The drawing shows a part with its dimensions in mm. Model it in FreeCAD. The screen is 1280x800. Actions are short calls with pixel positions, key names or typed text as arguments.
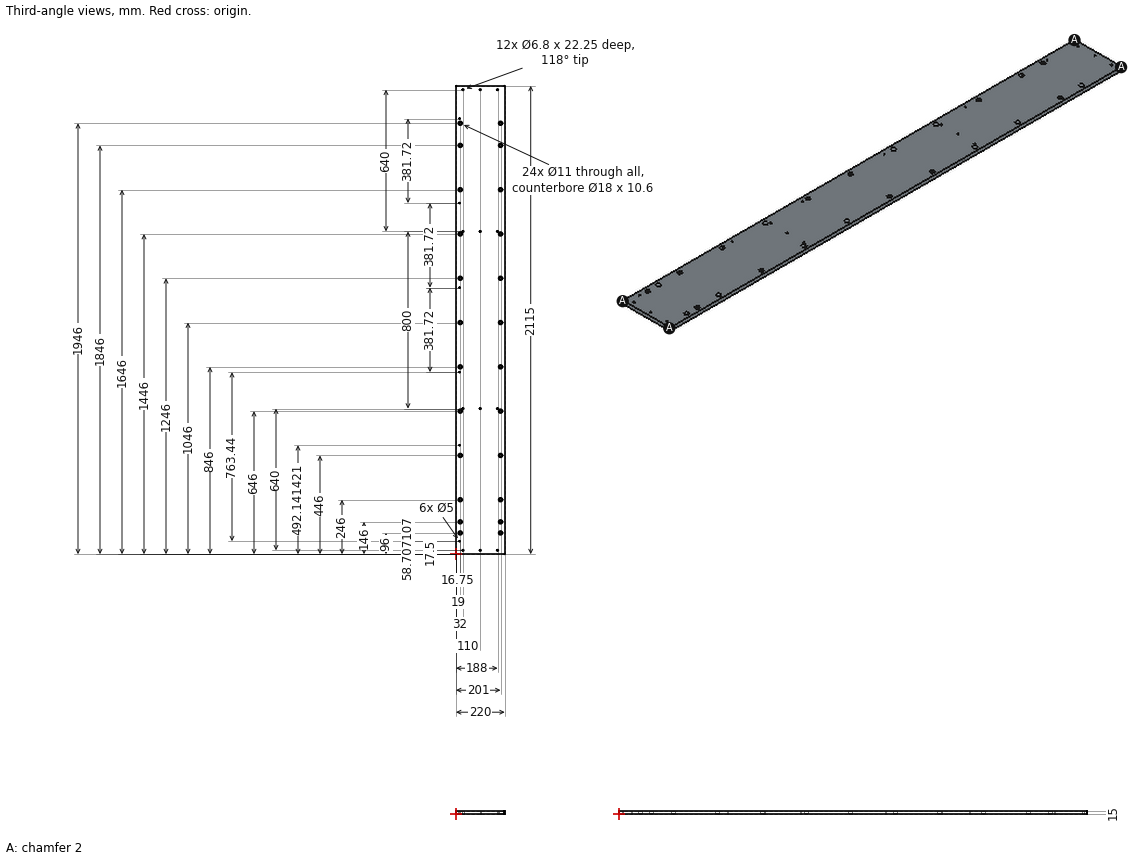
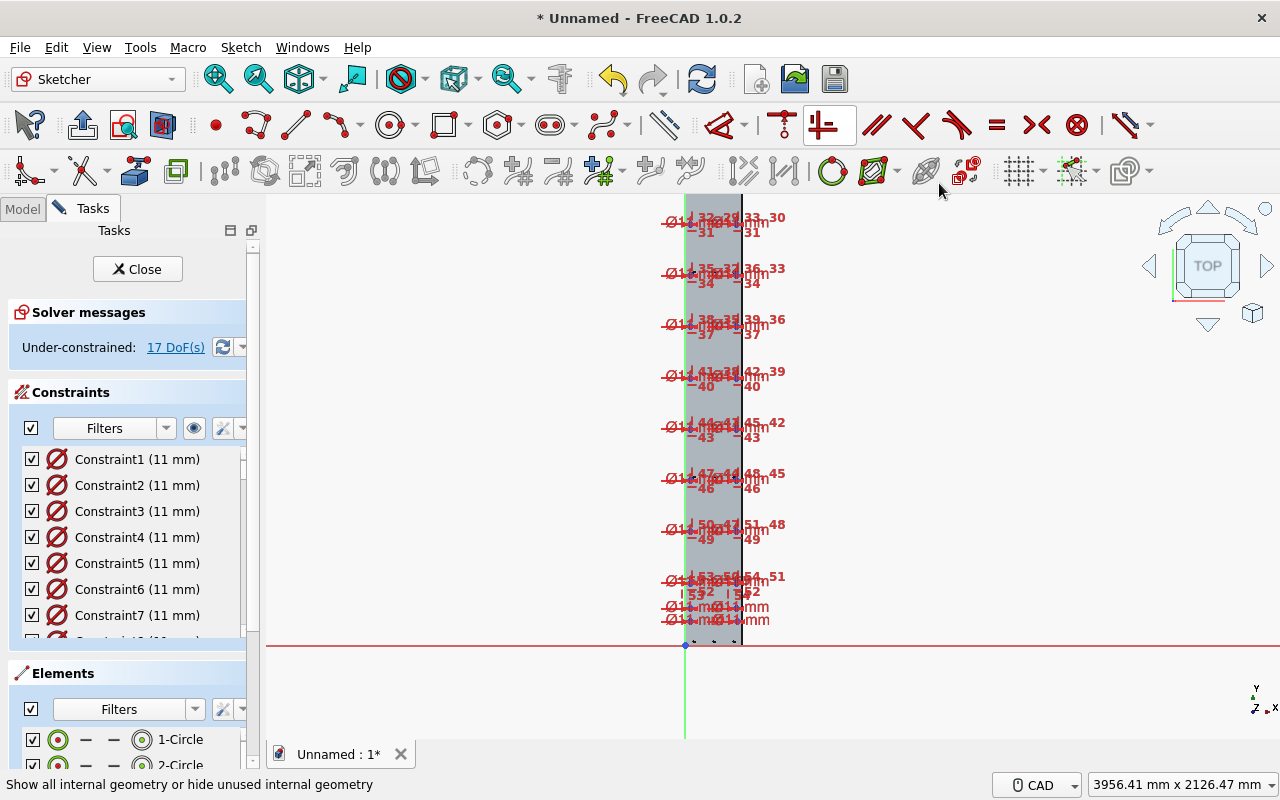
click(690, 609)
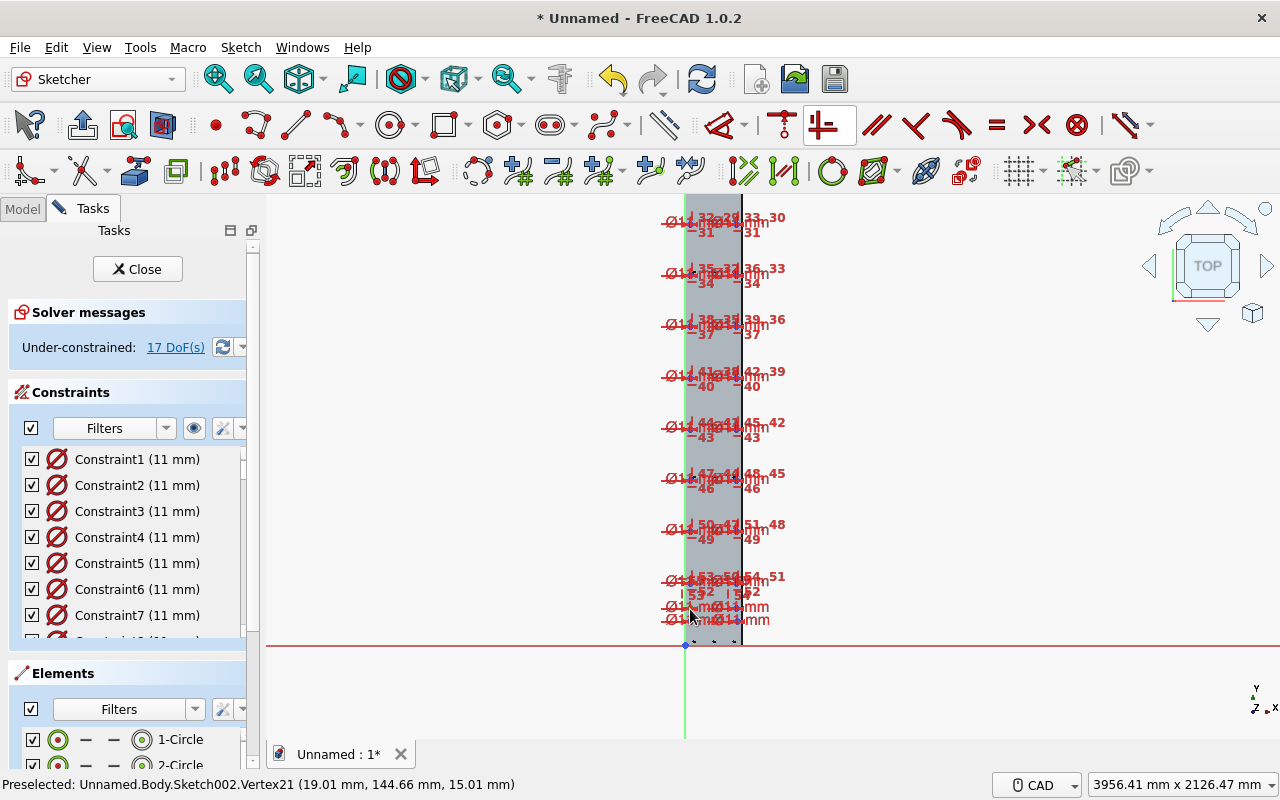
click(690, 622)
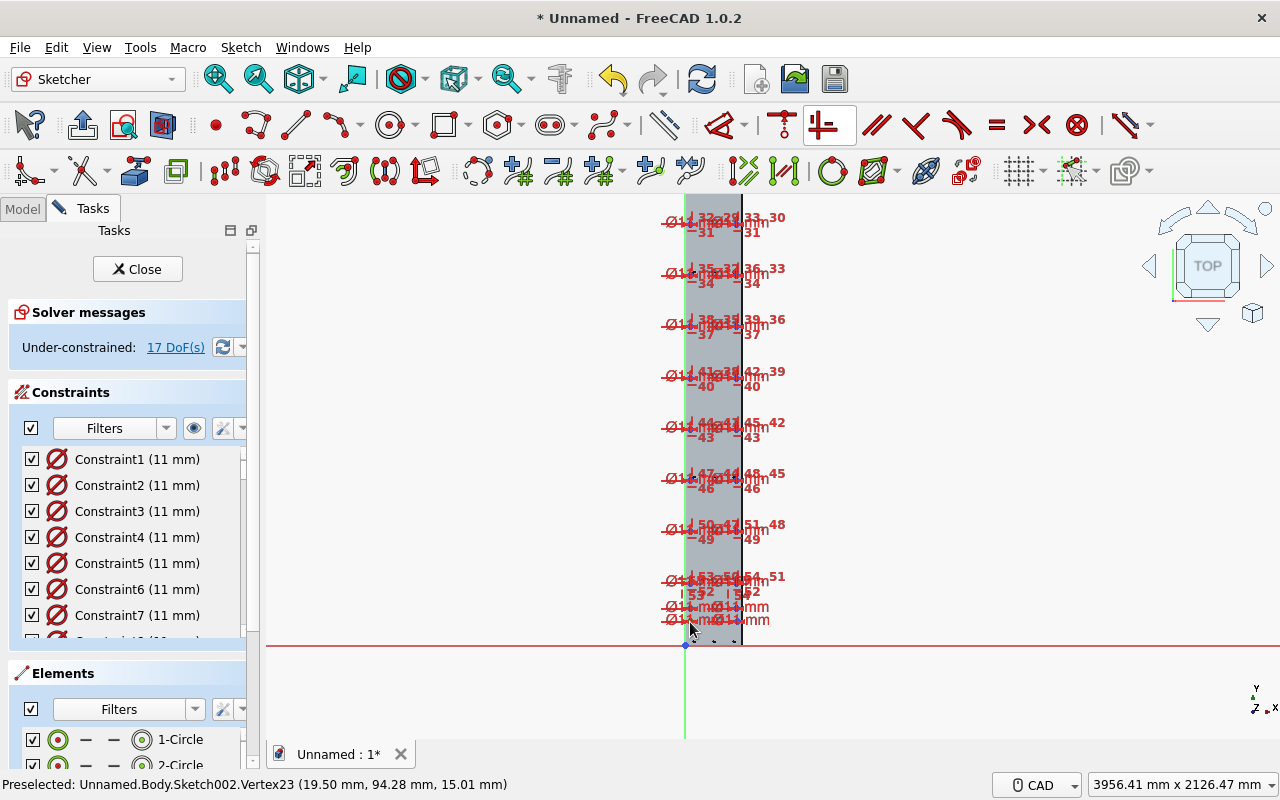
key(v)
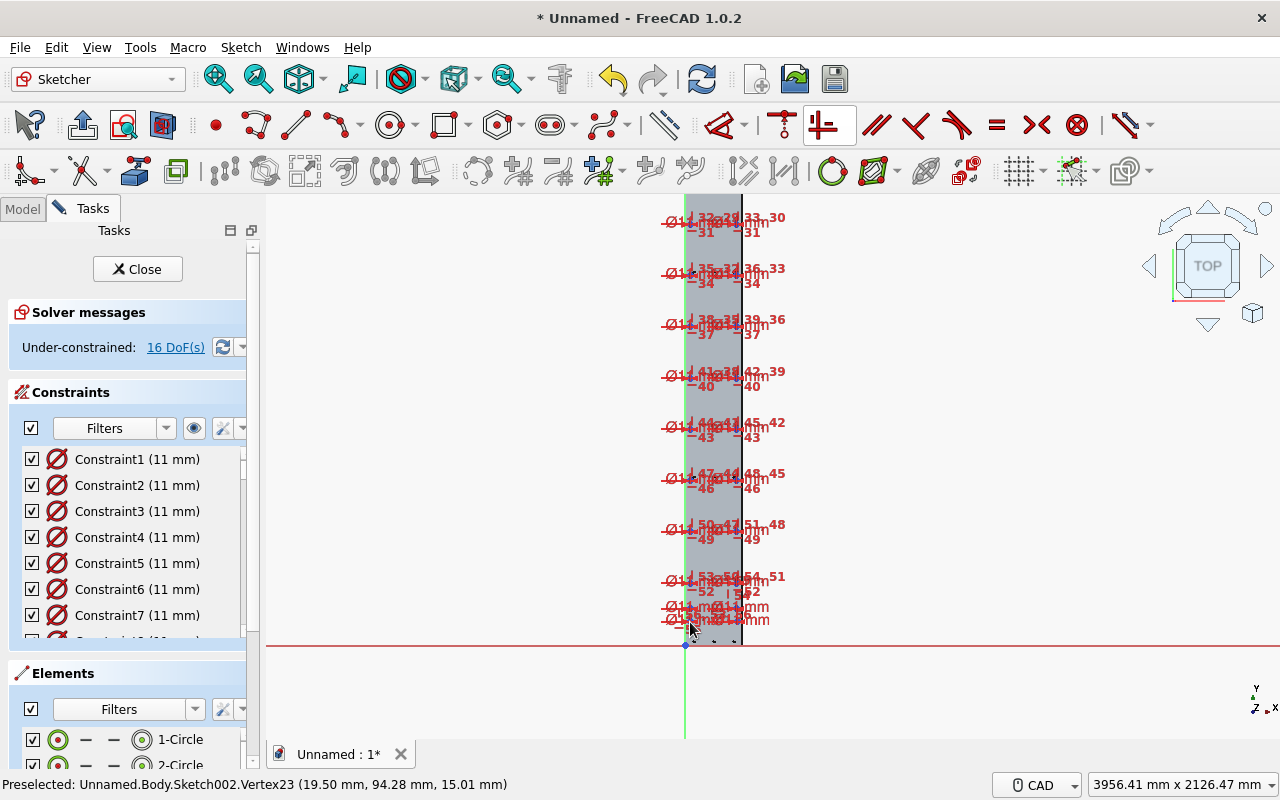
scroll(736, 609, up, 4)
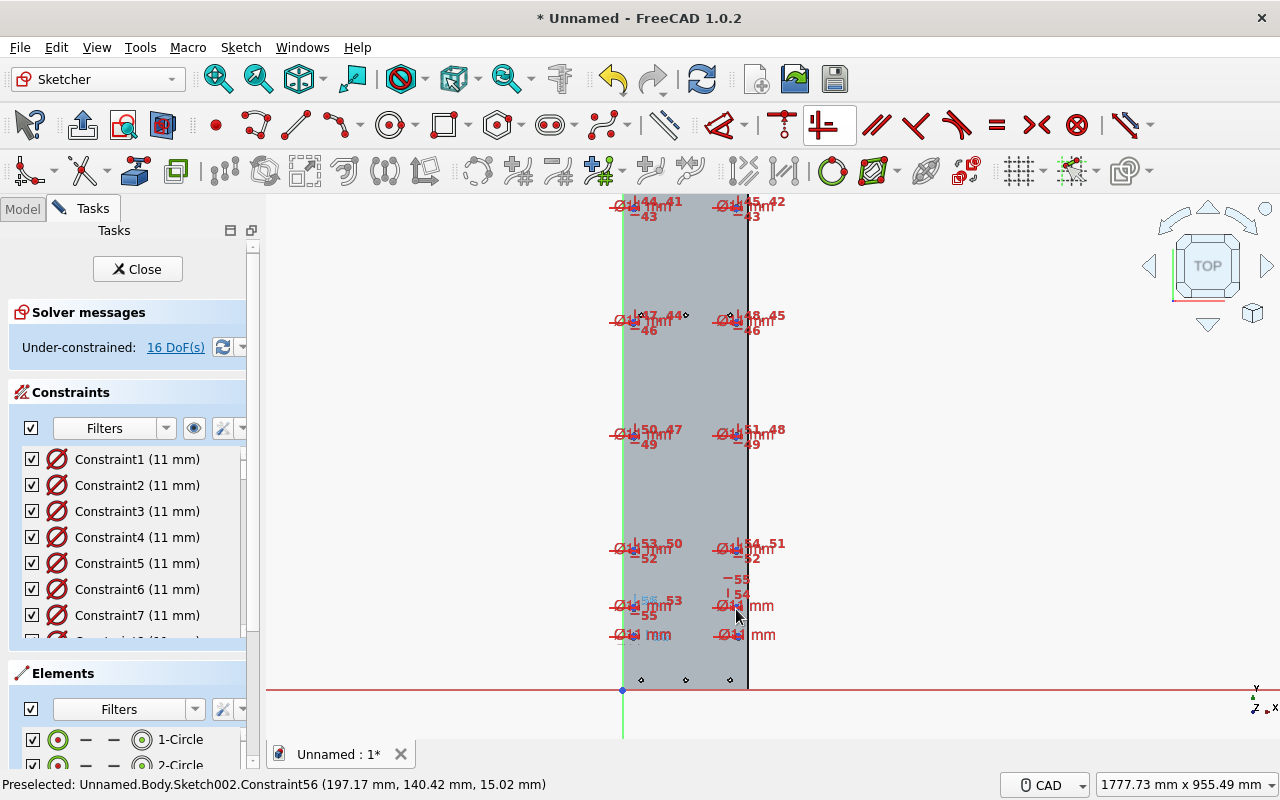
click(737, 608)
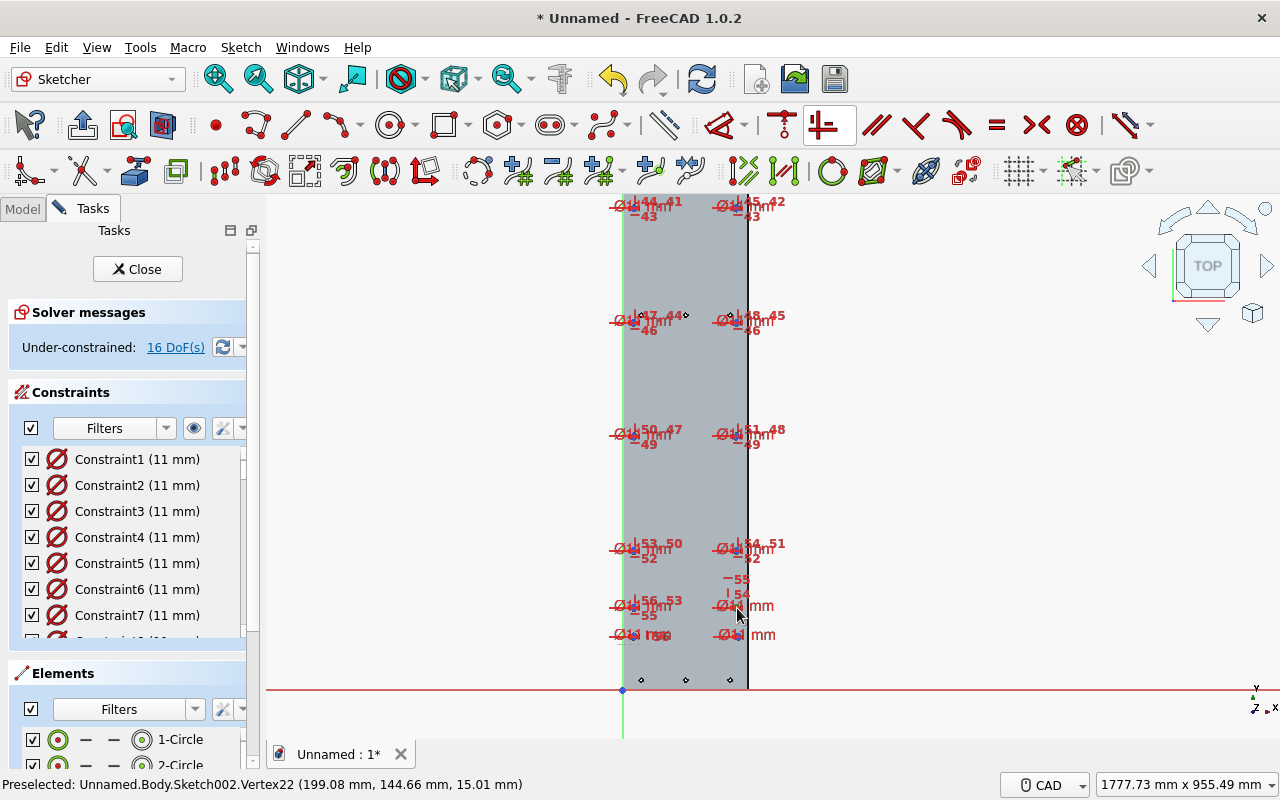
click(738, 637)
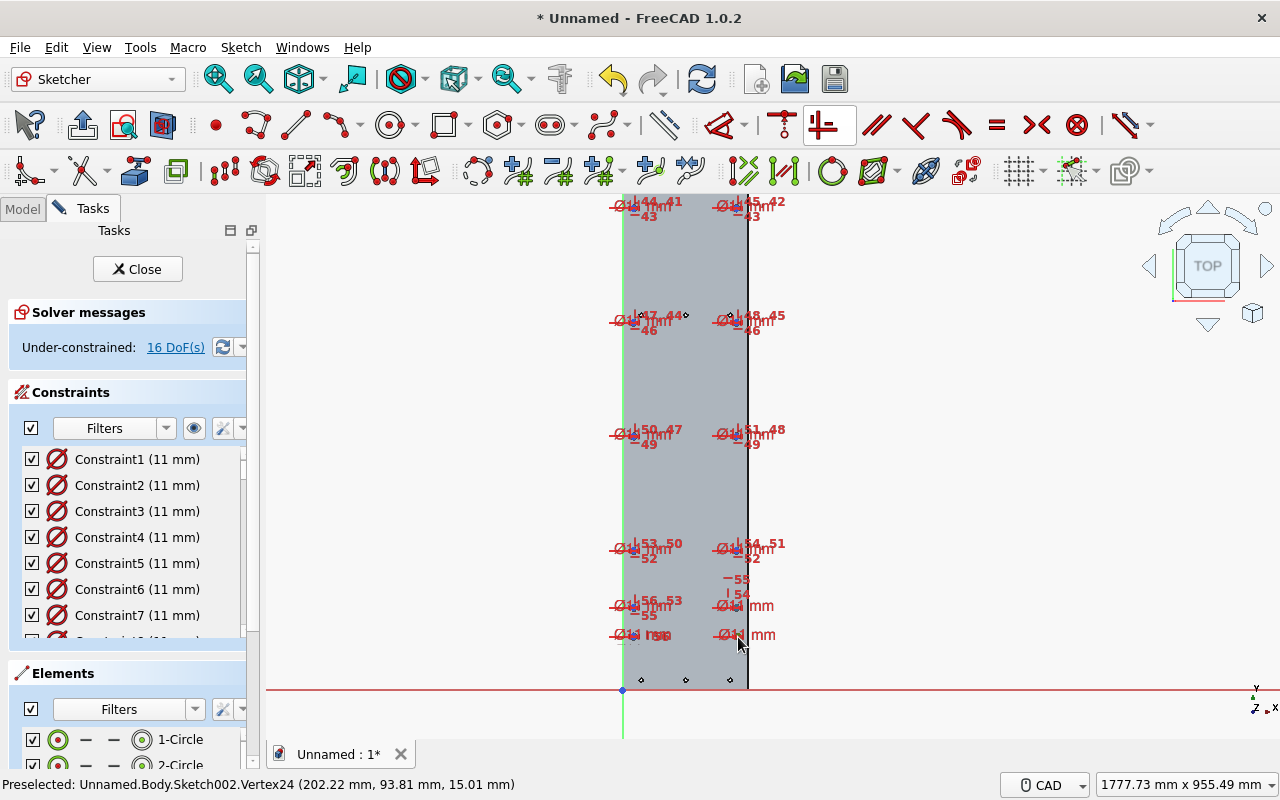
key(v)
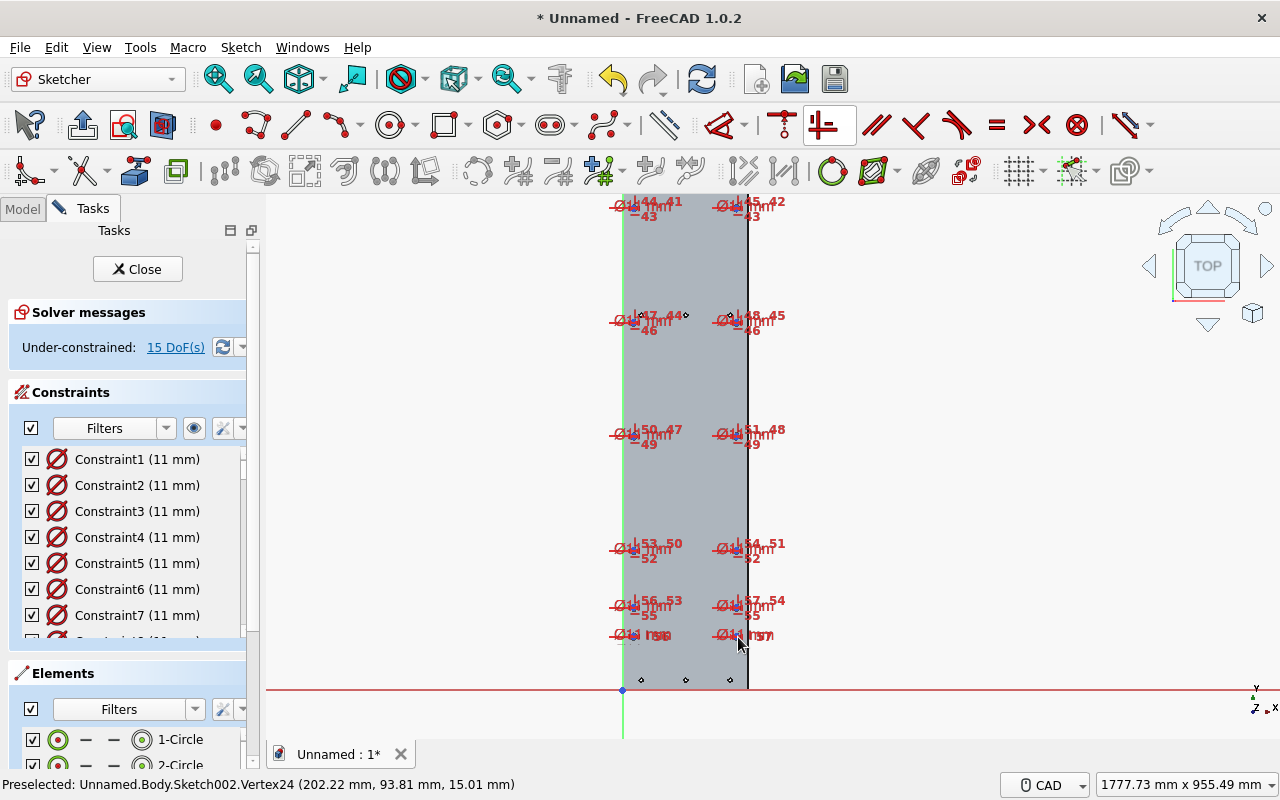
click(634, 637)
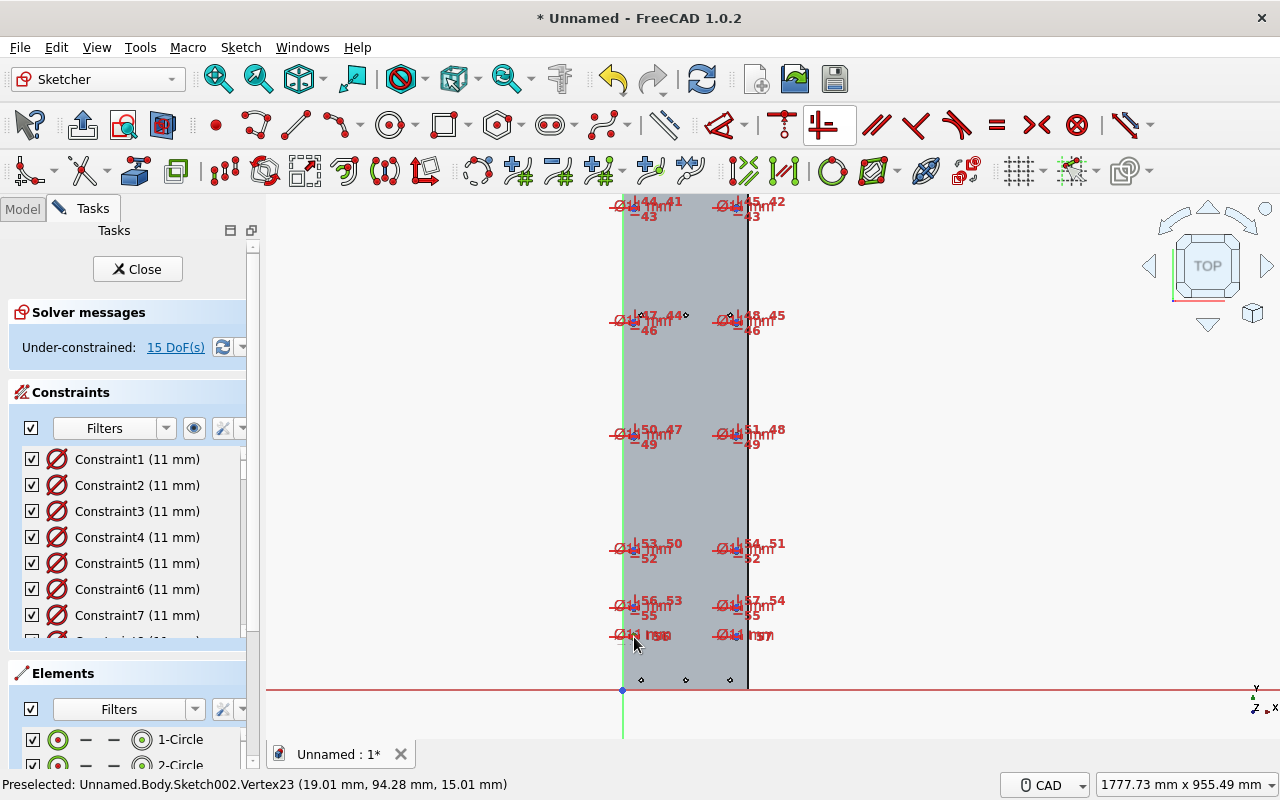
click(737, 637)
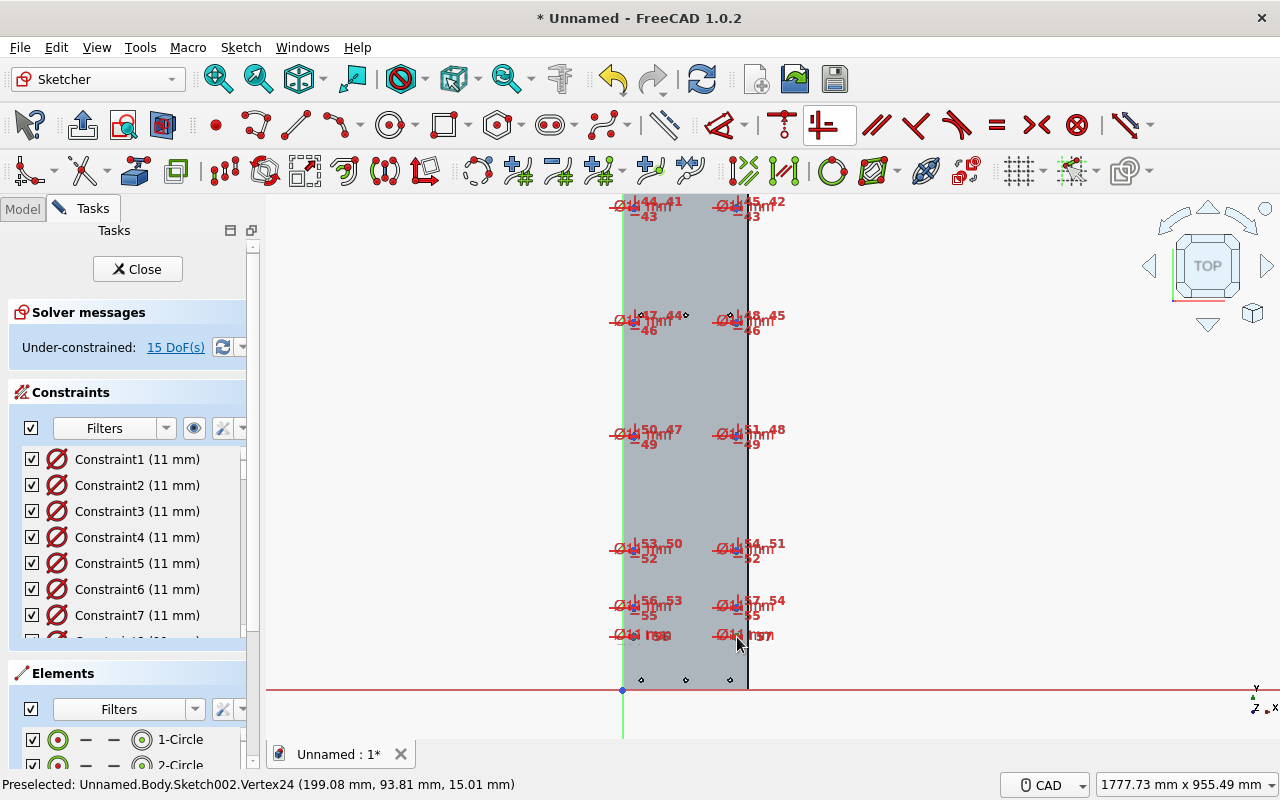
key(h)